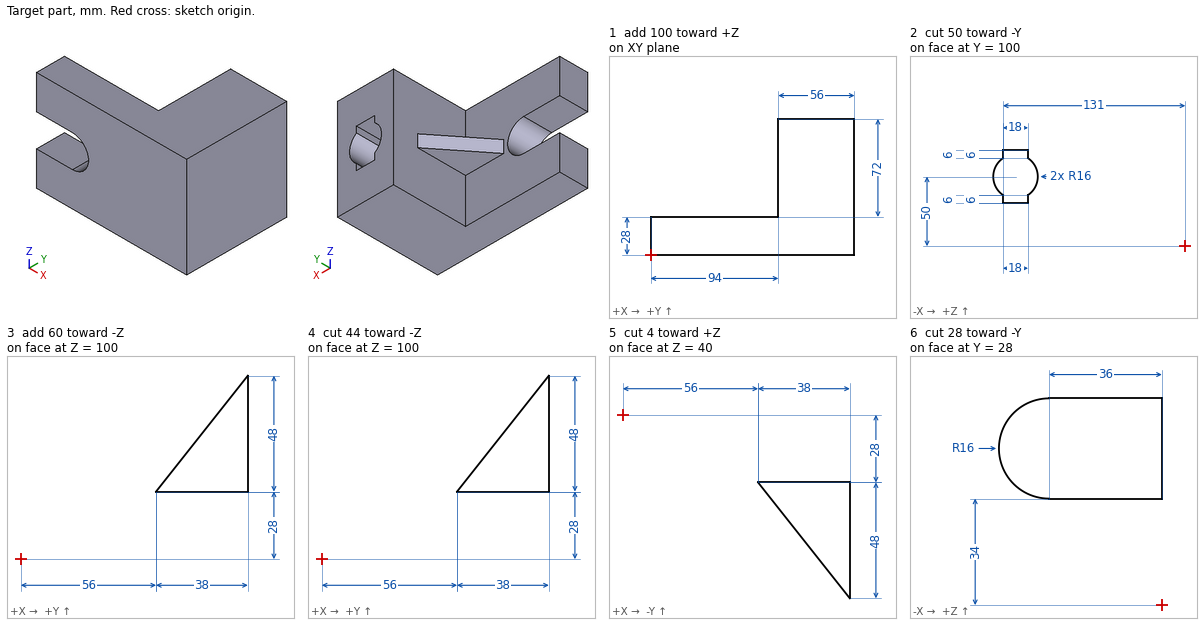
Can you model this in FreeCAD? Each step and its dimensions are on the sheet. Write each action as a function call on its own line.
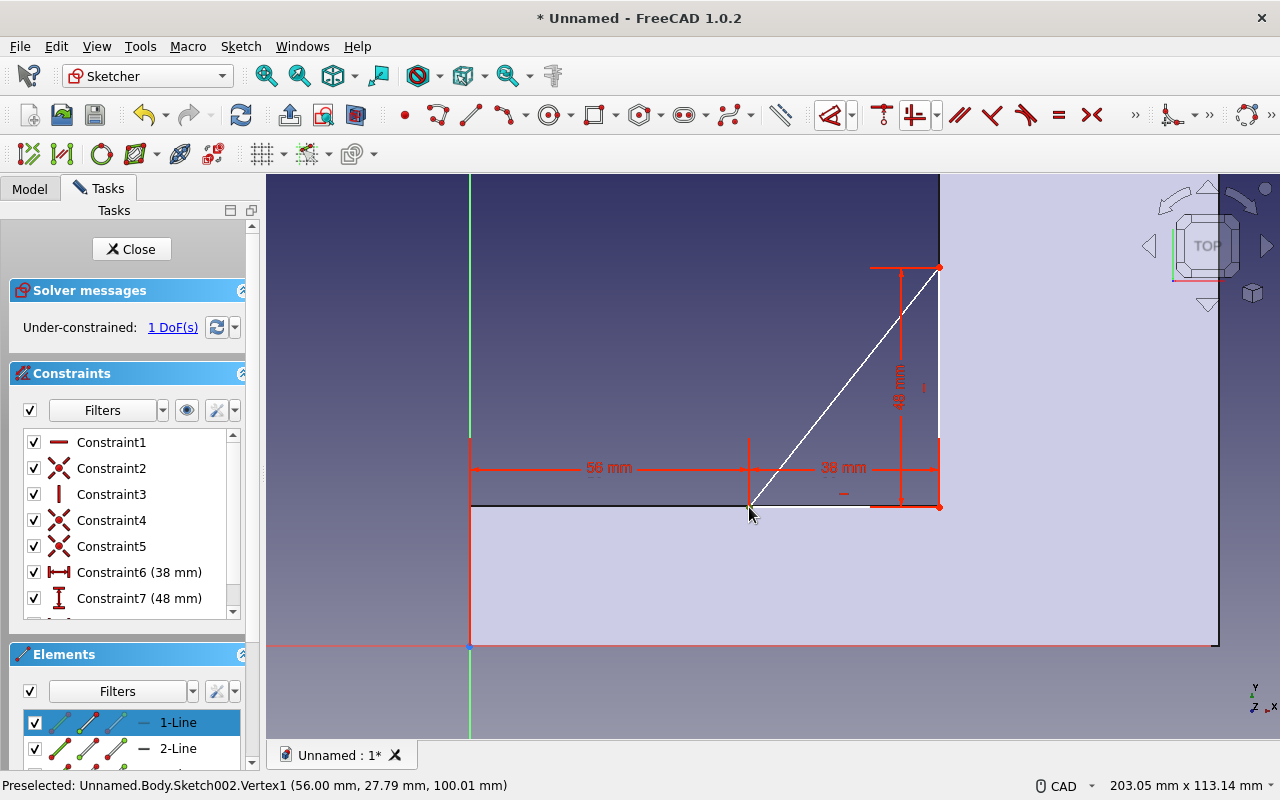
click(852, 116)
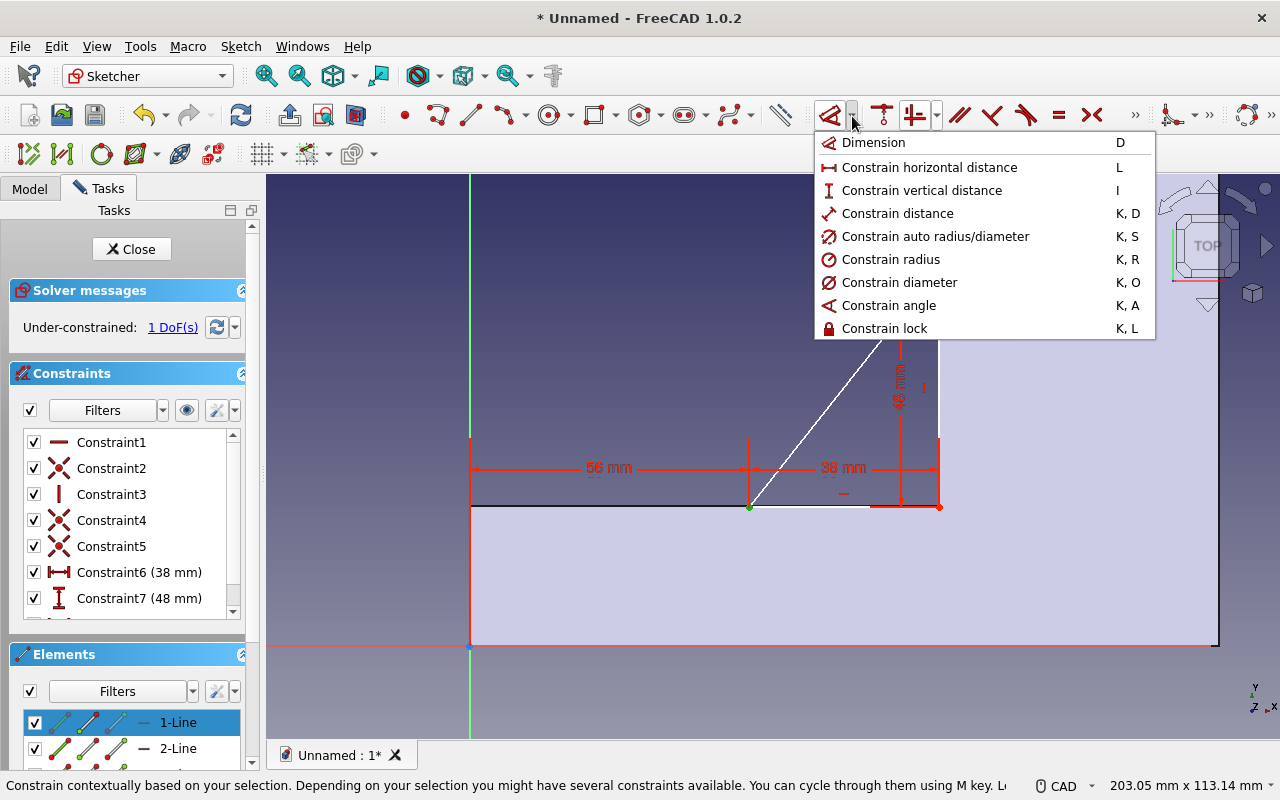
click(985, 190)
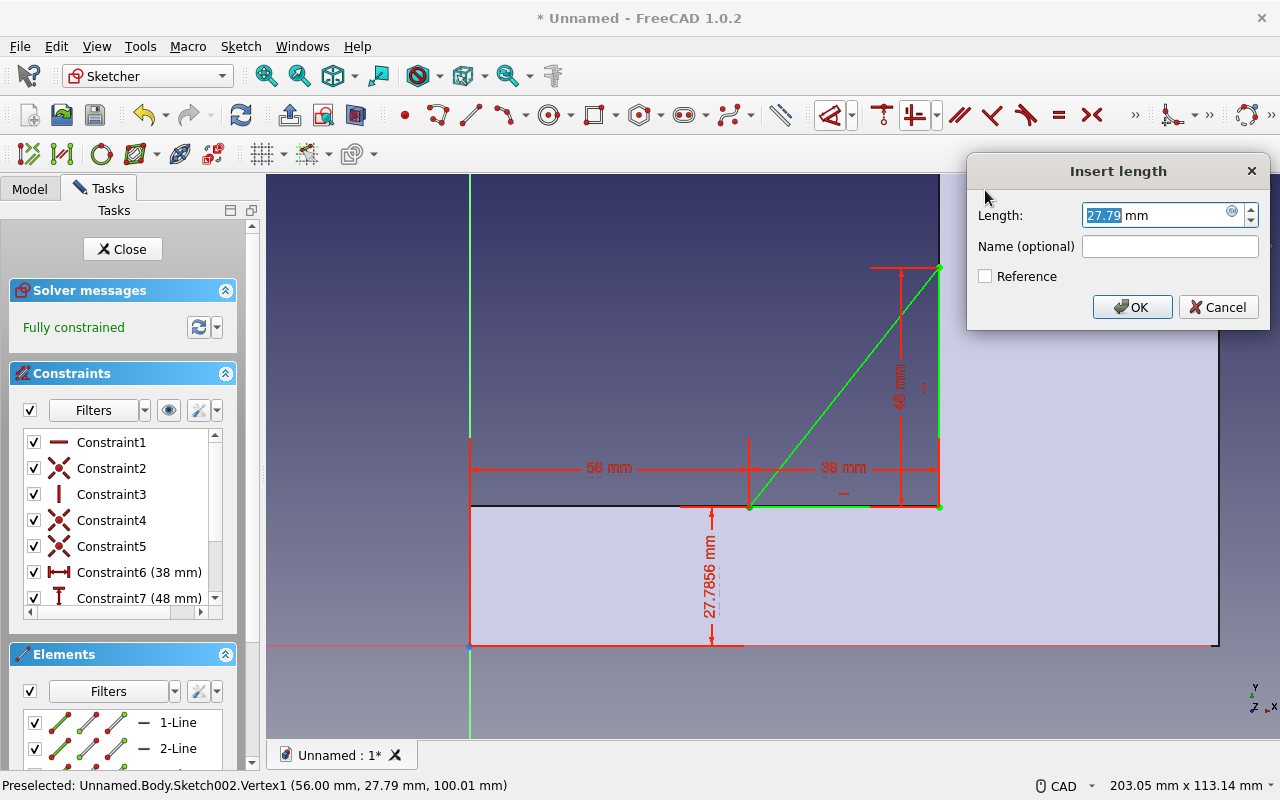
text(28)
key(Return)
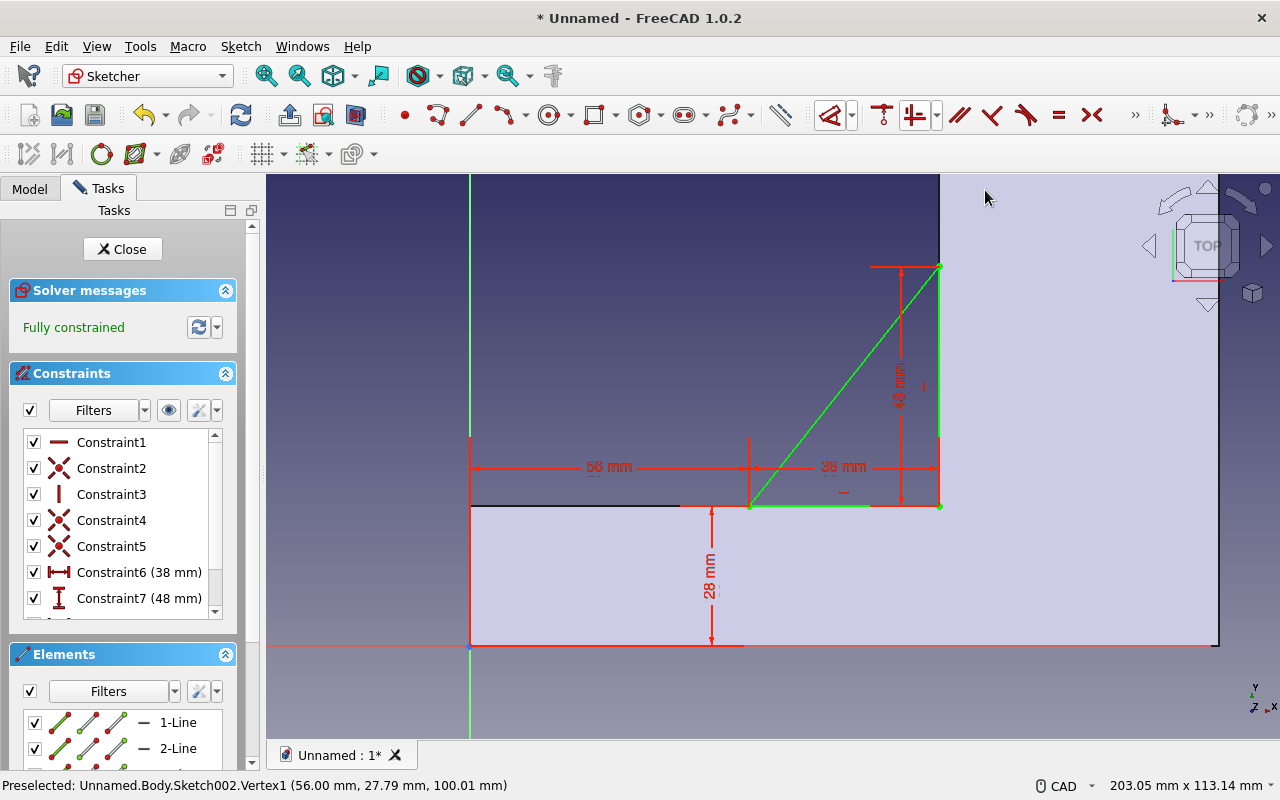
click(123, 249)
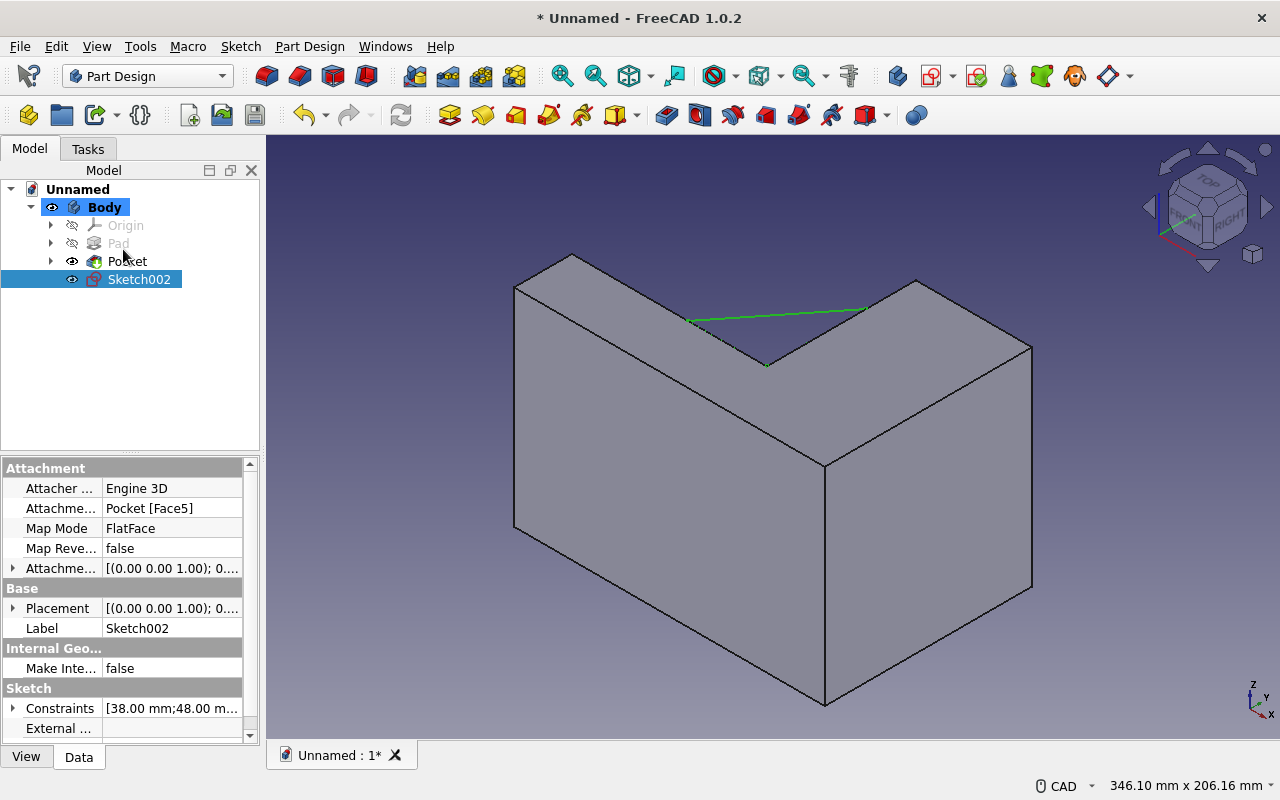
click(450, 116)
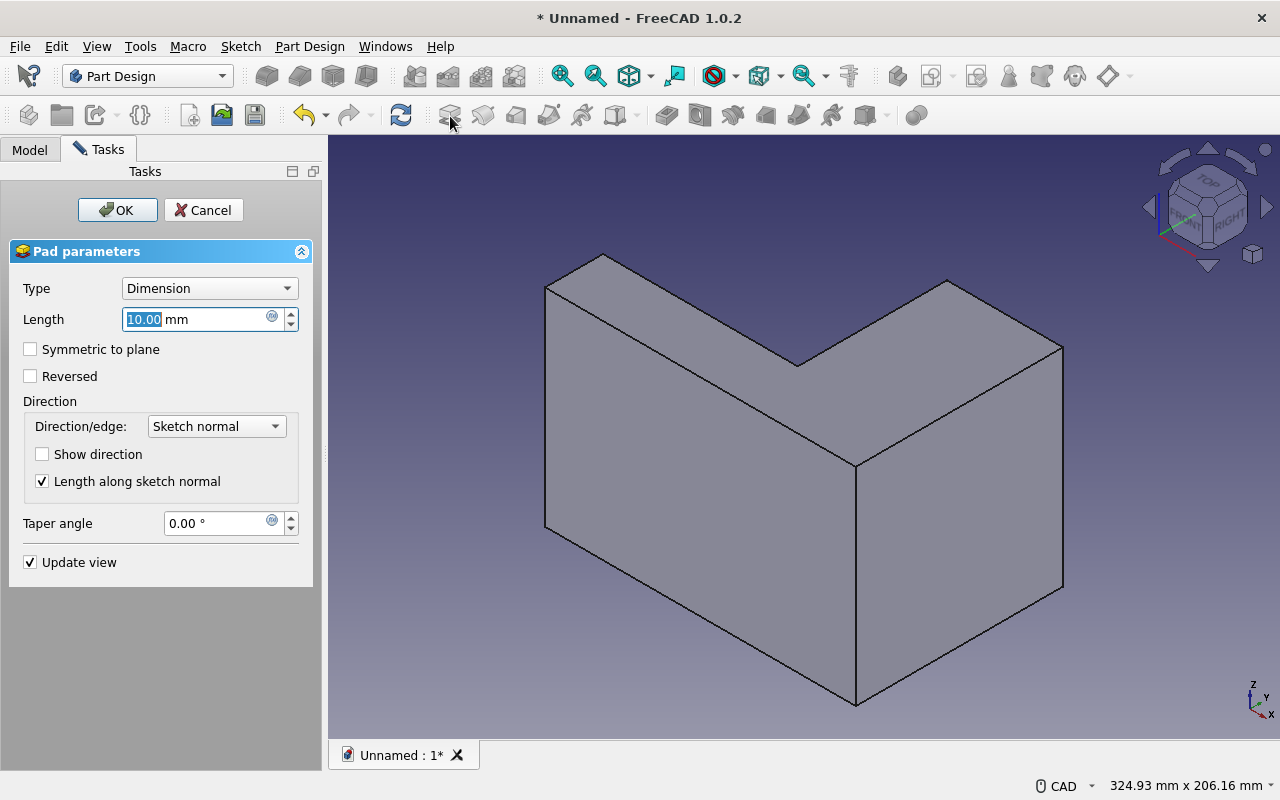
text(60)
key(Tab)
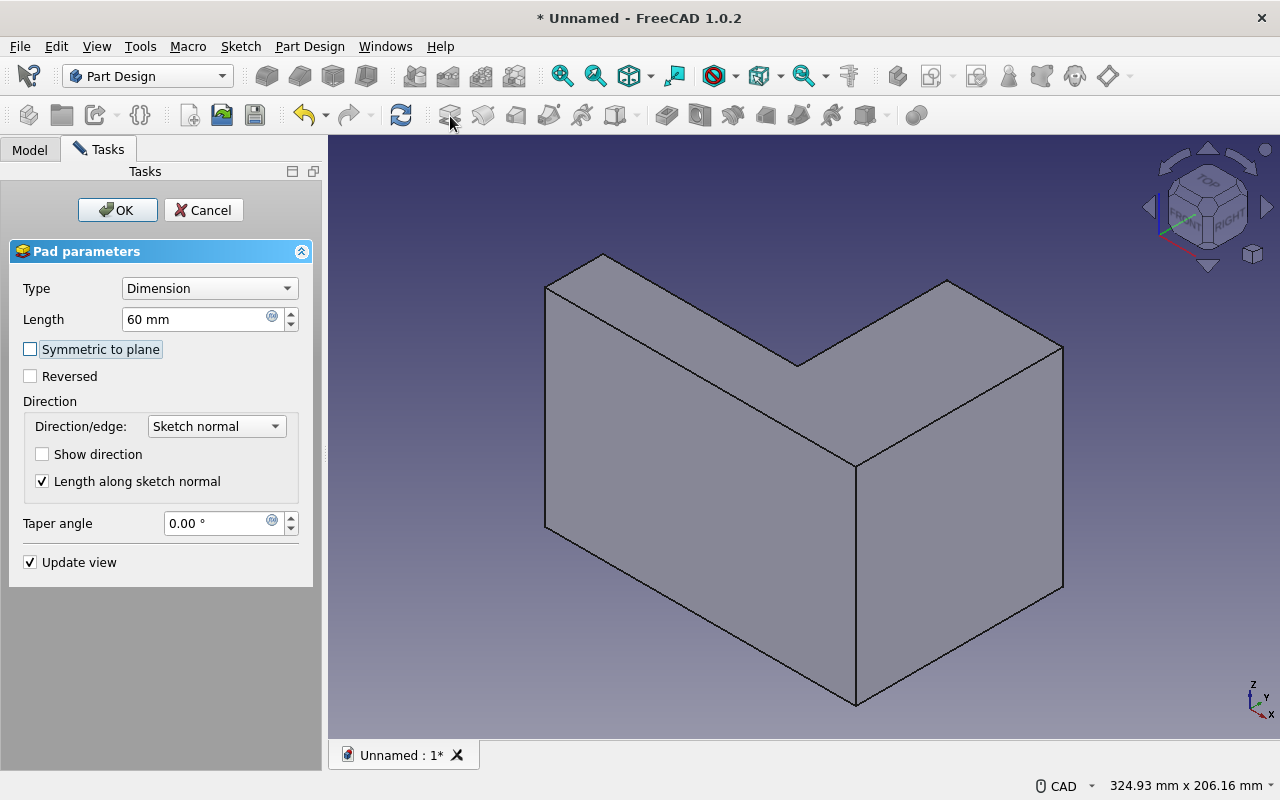
click(31, 376)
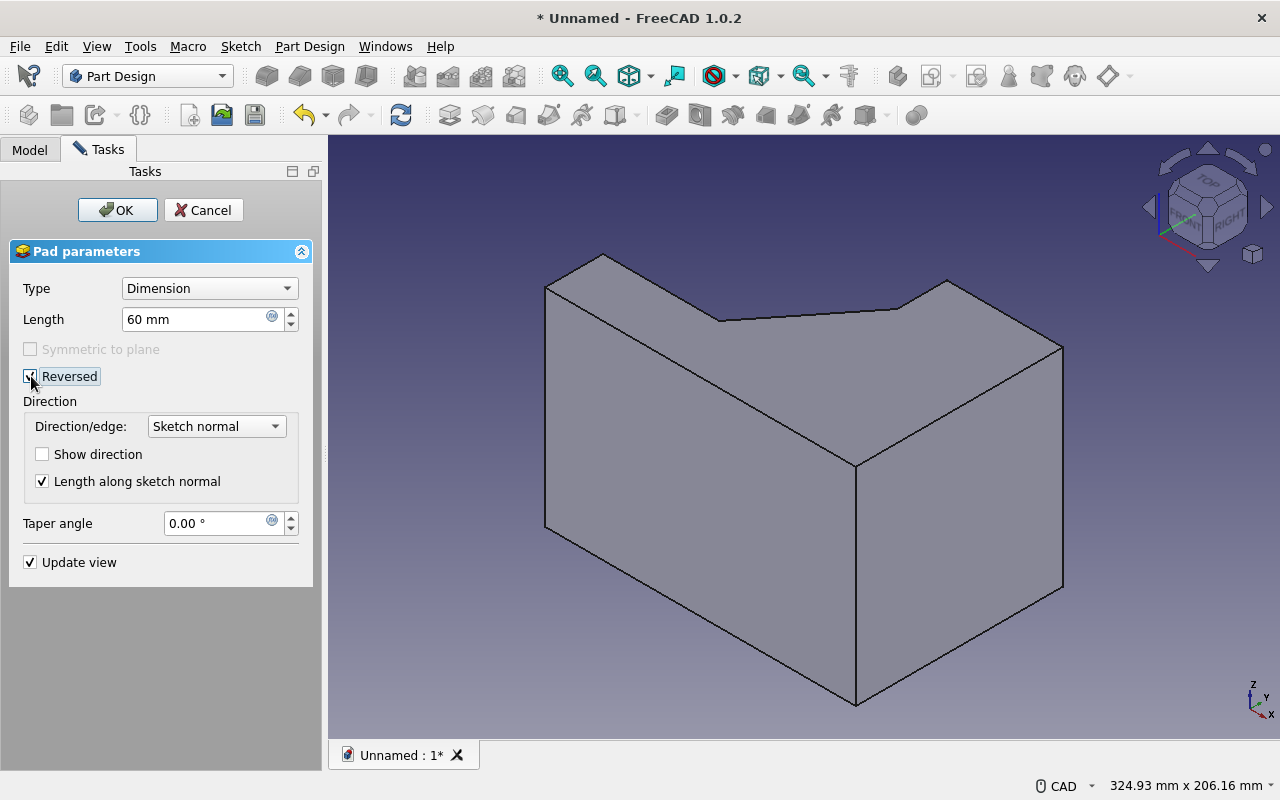
click(118, 210)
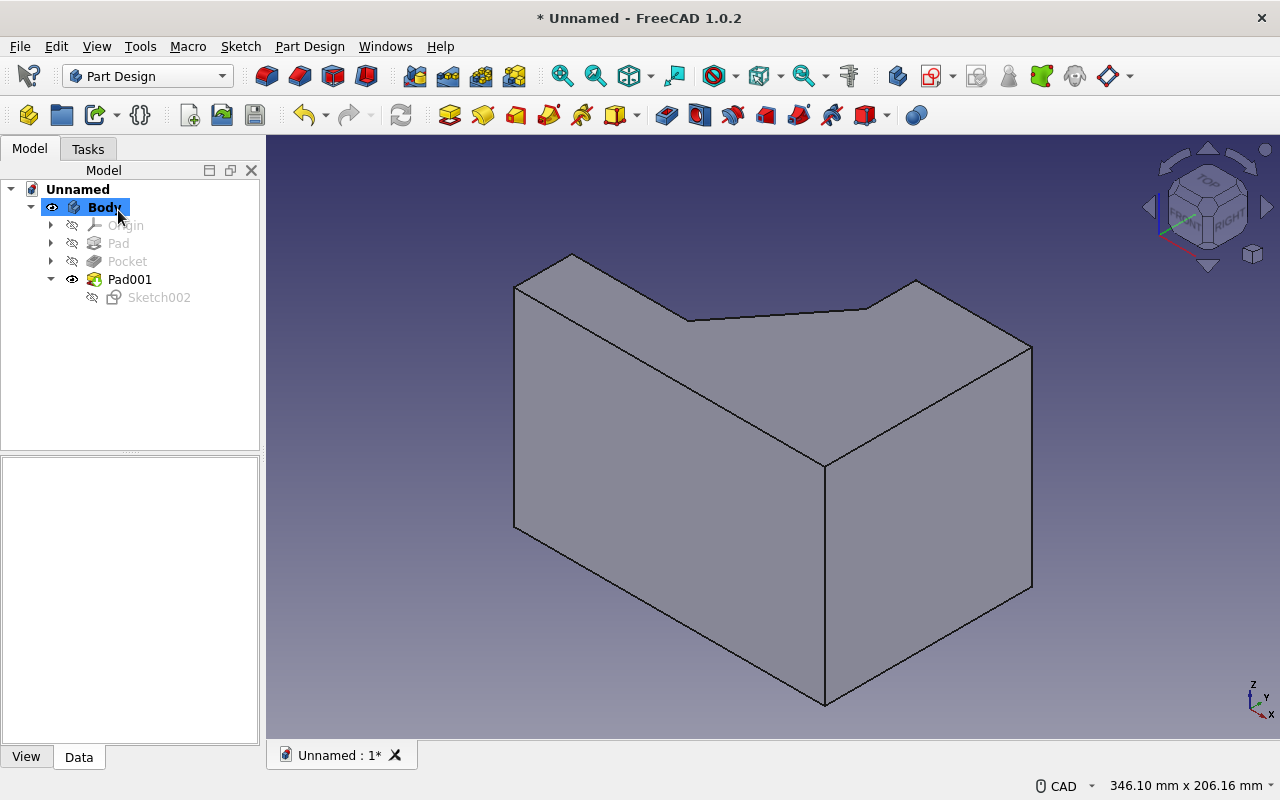
click(862, 368)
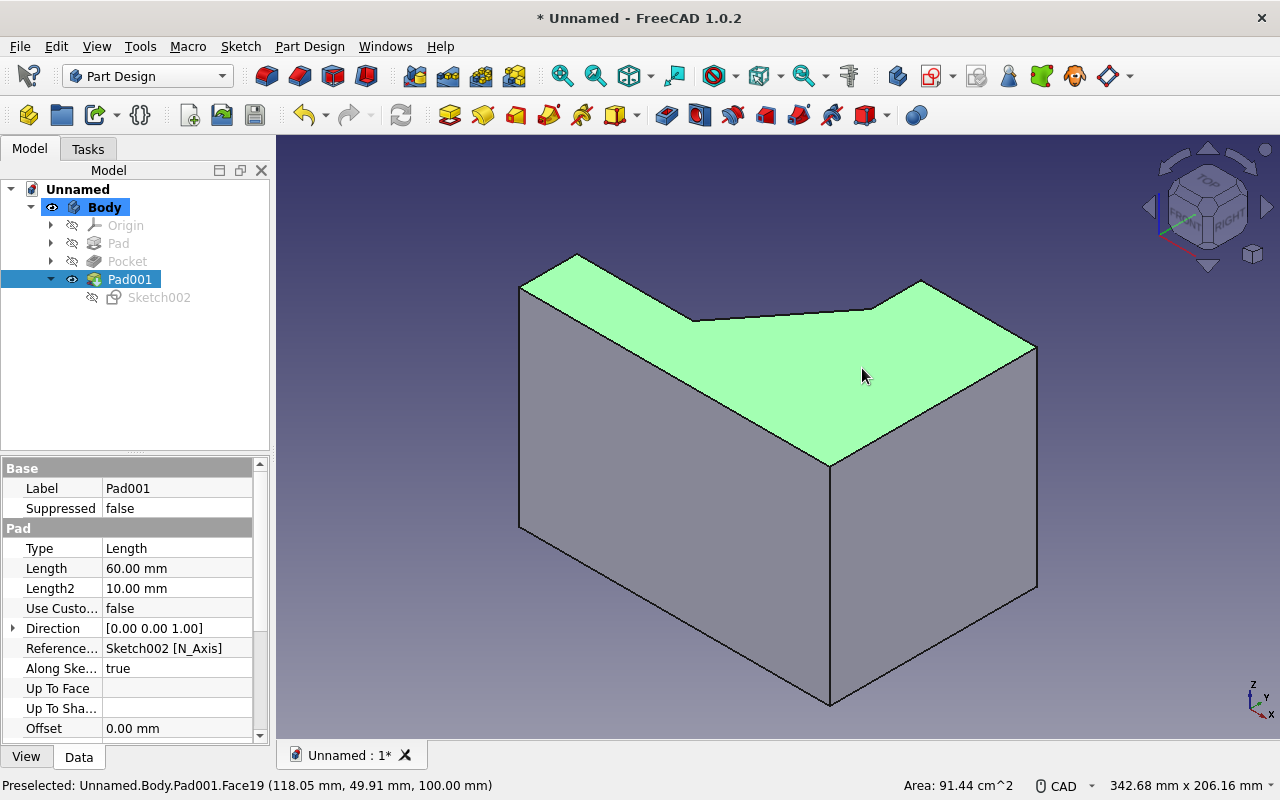
click(930, 76)